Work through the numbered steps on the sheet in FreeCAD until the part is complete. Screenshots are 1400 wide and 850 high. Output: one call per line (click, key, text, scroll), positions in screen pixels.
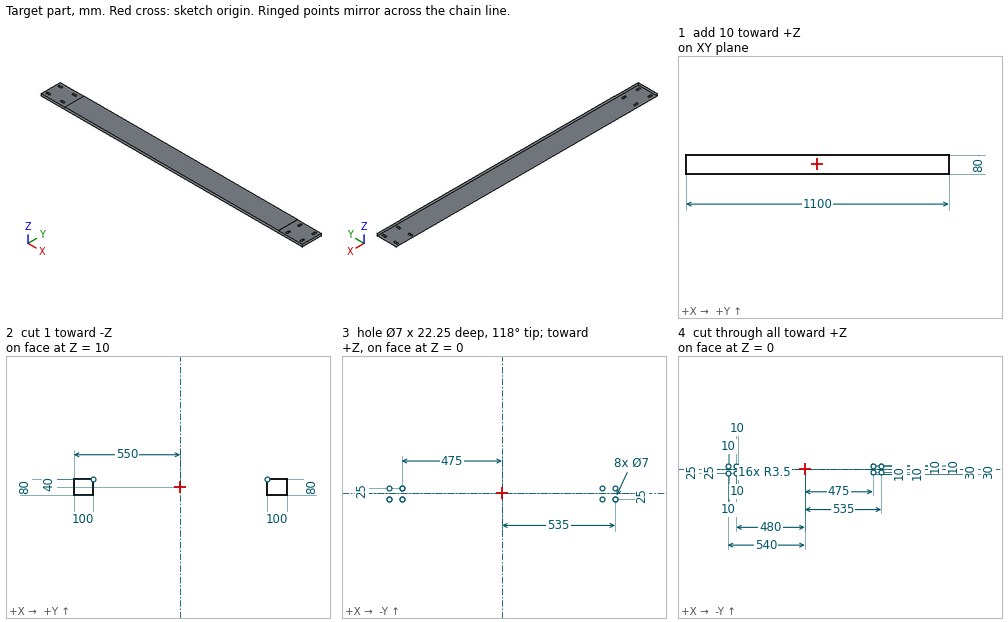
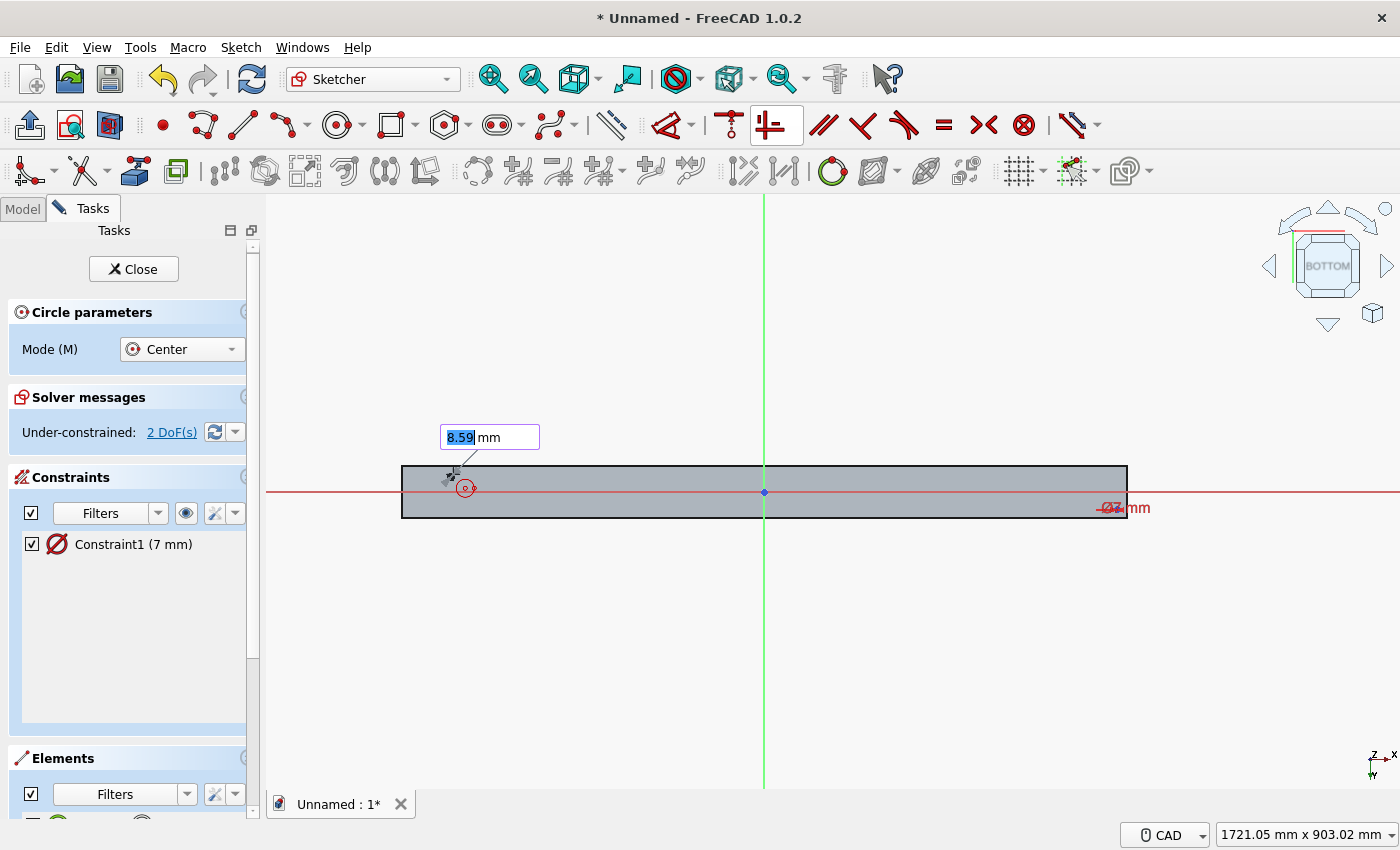
text(7)
key(Return)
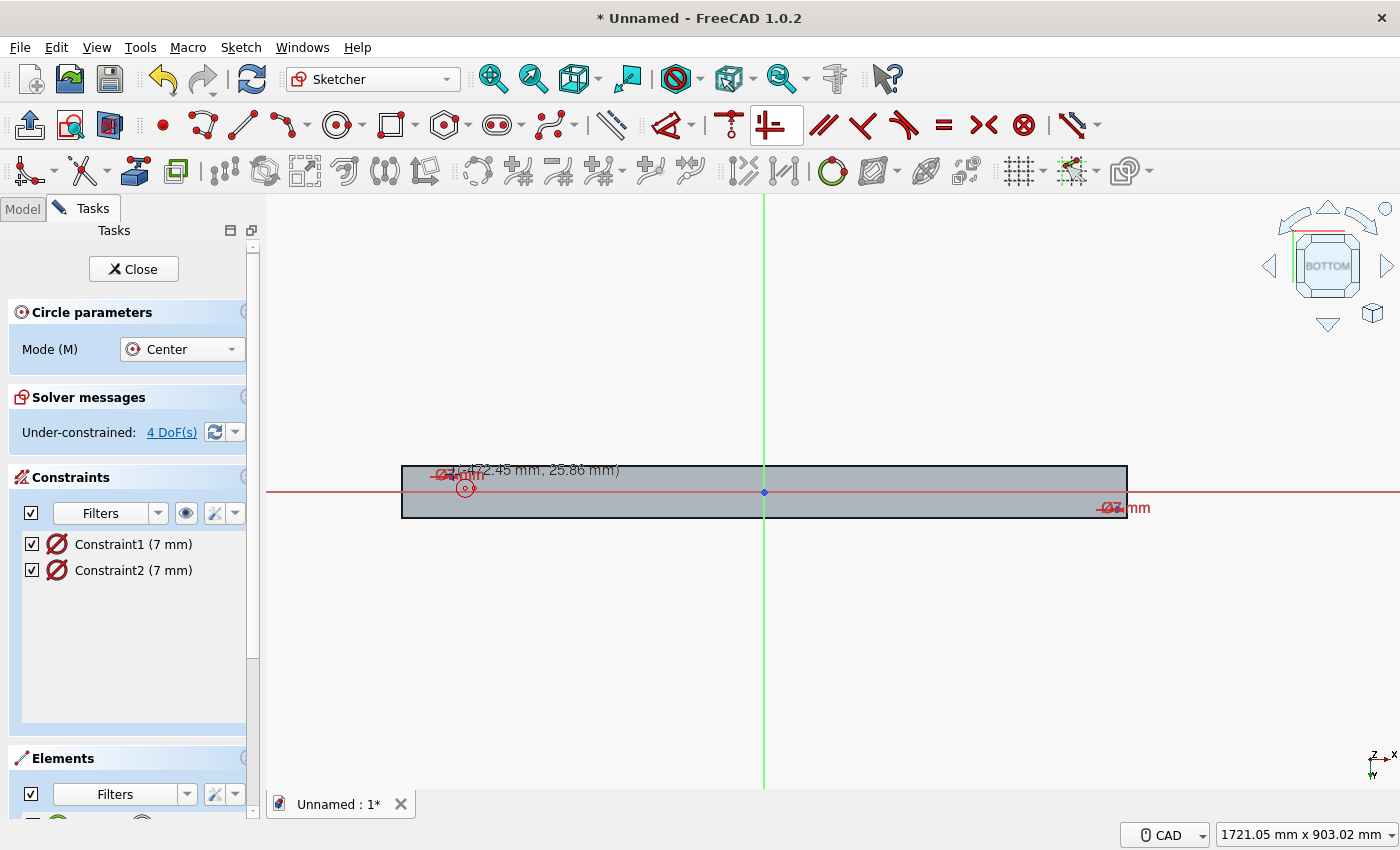
scroll(412, 509, up, 12)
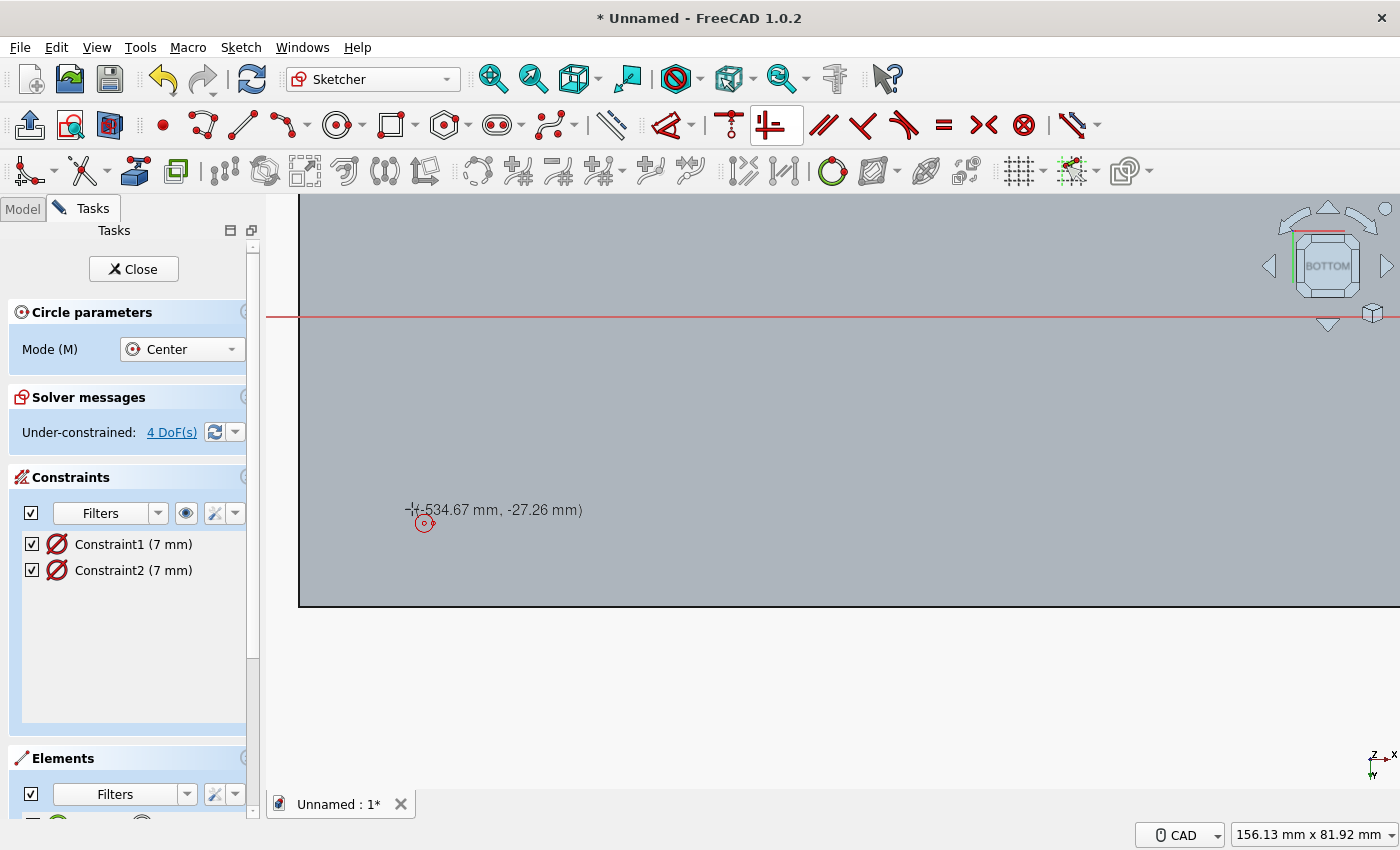
scroll(412, 509, down, 12)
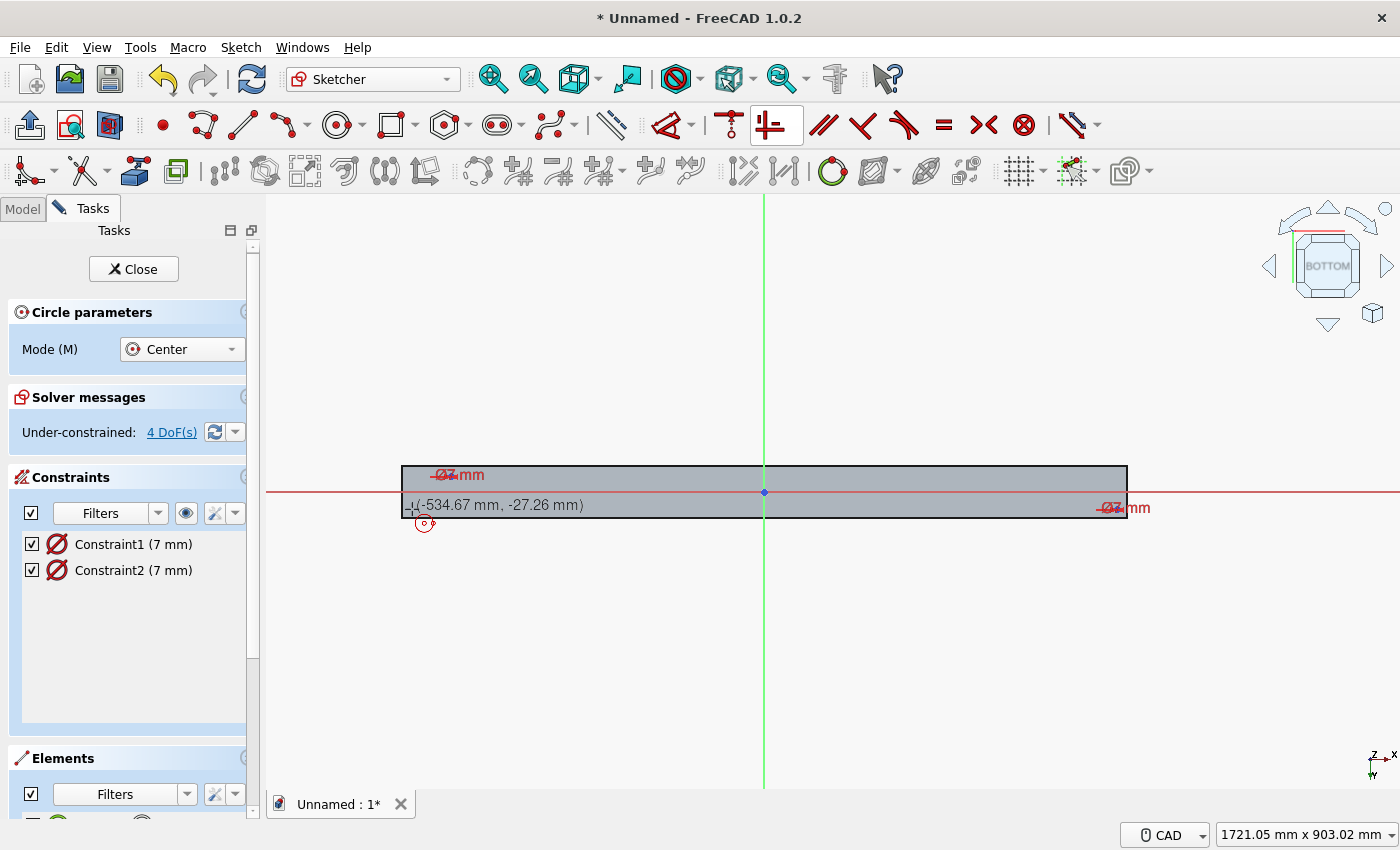
click(412, 509)
move(413, 507)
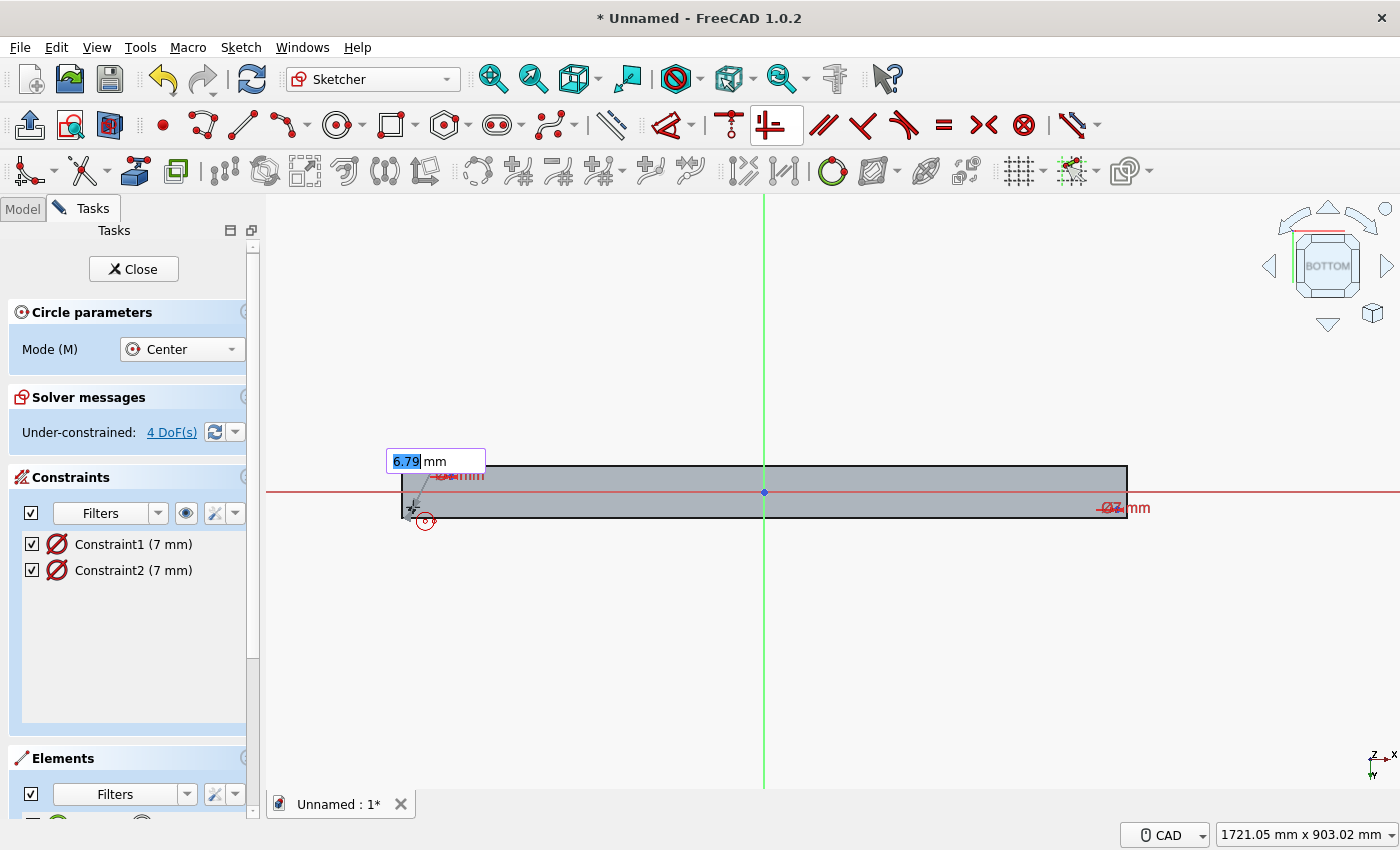
text(7)
key(Return)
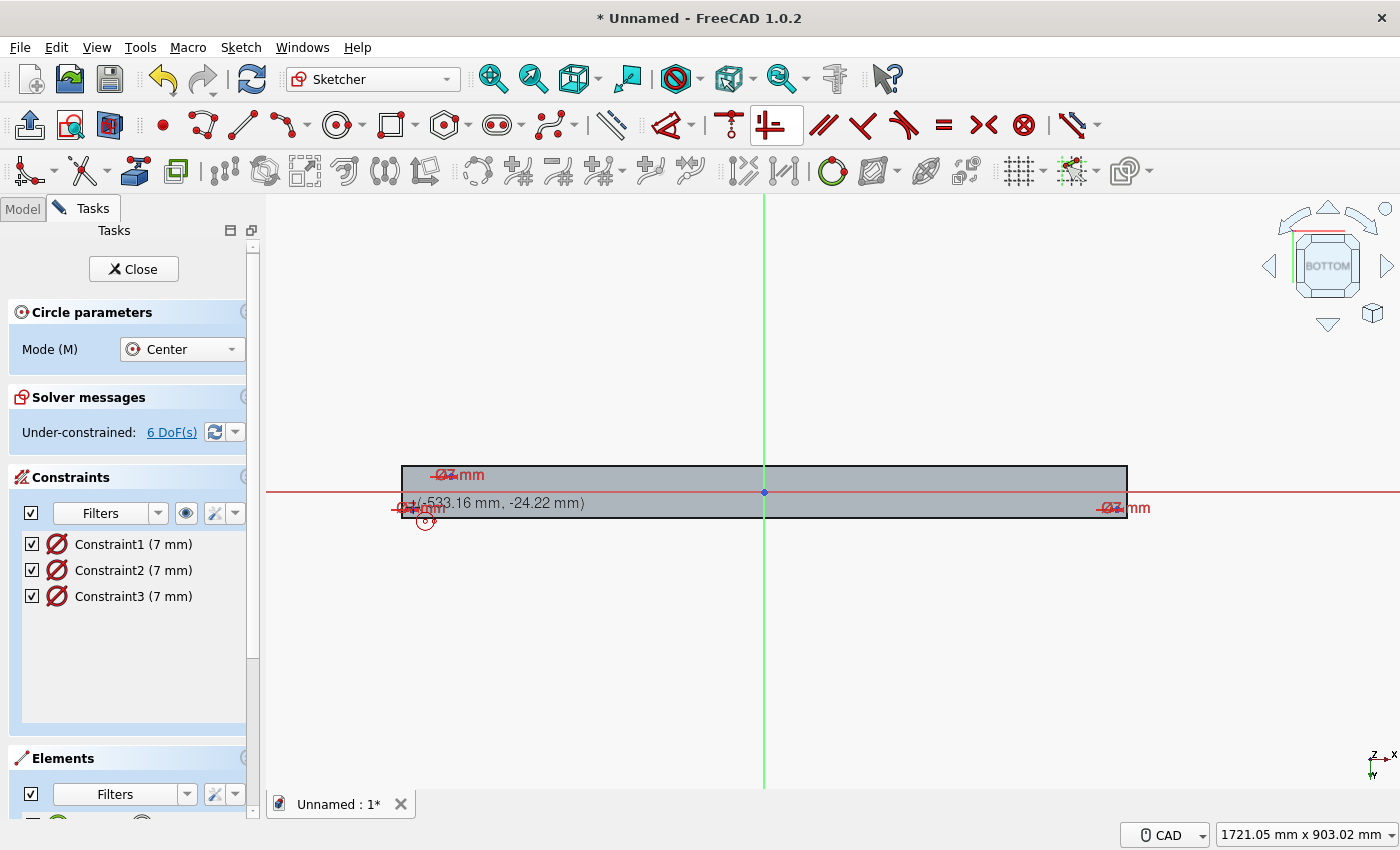
scroll(412, 476, up, 12)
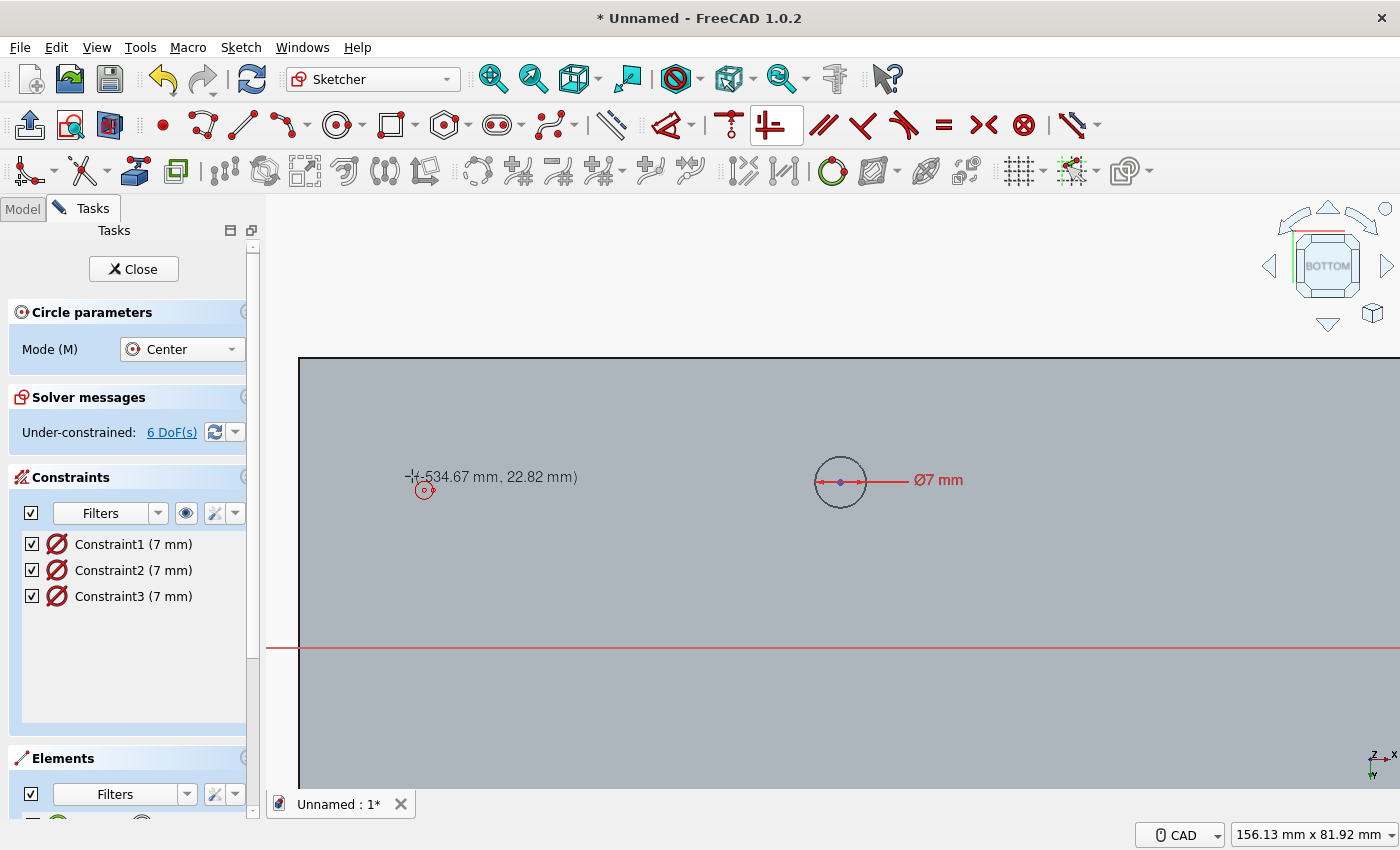
scroll(412, 476, down, 12)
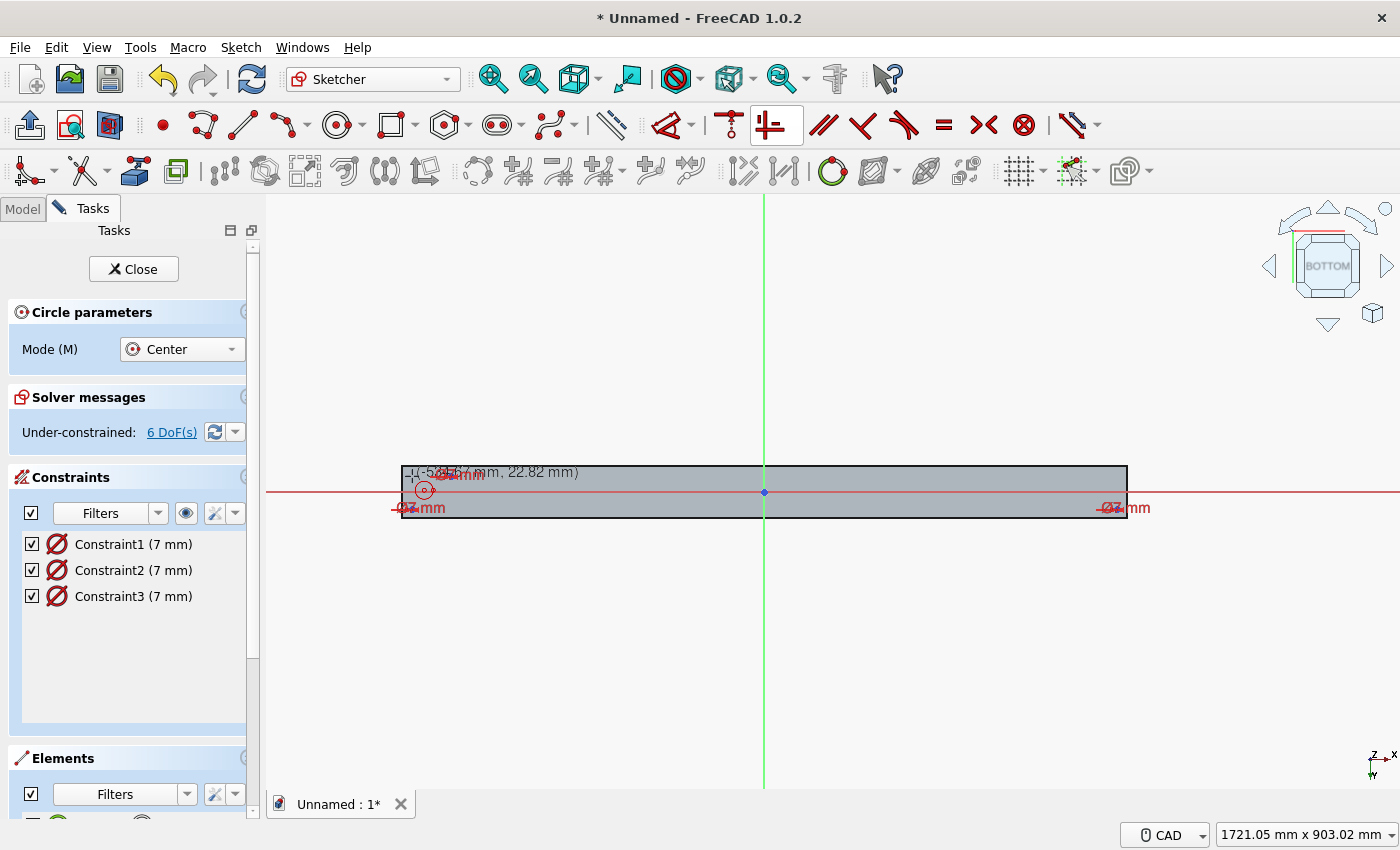
click(412, 476)
move(413, 474)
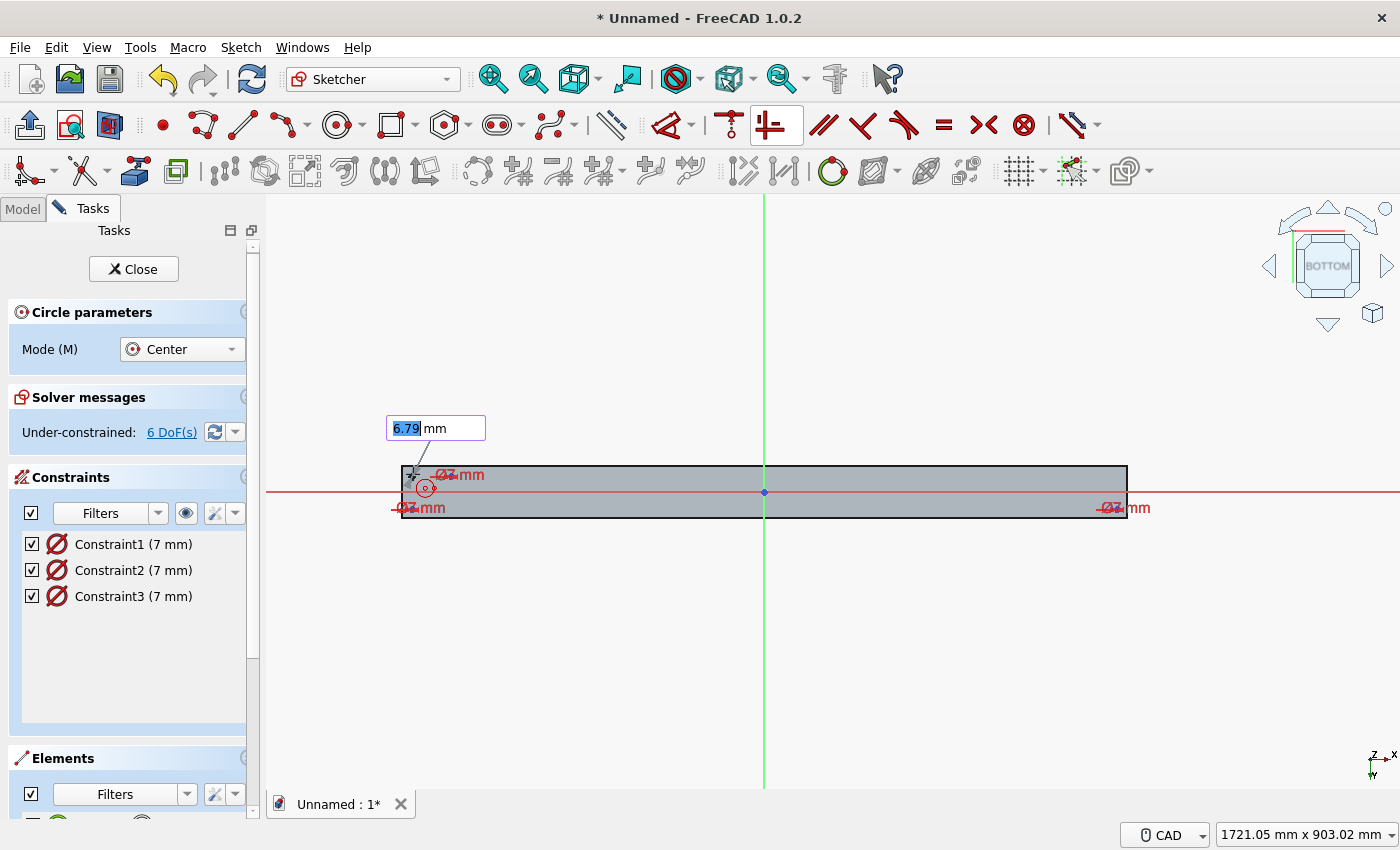
text(7)
key(Return)